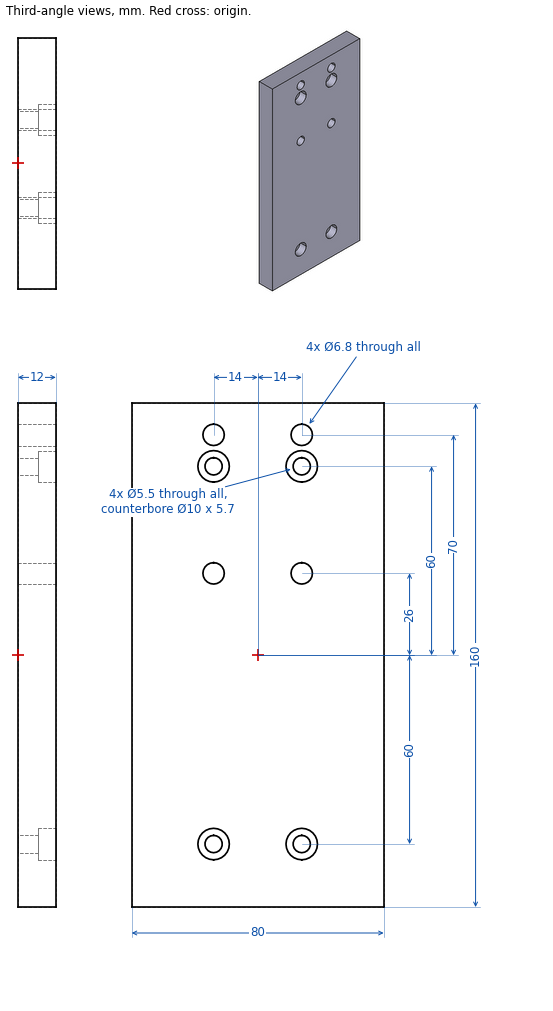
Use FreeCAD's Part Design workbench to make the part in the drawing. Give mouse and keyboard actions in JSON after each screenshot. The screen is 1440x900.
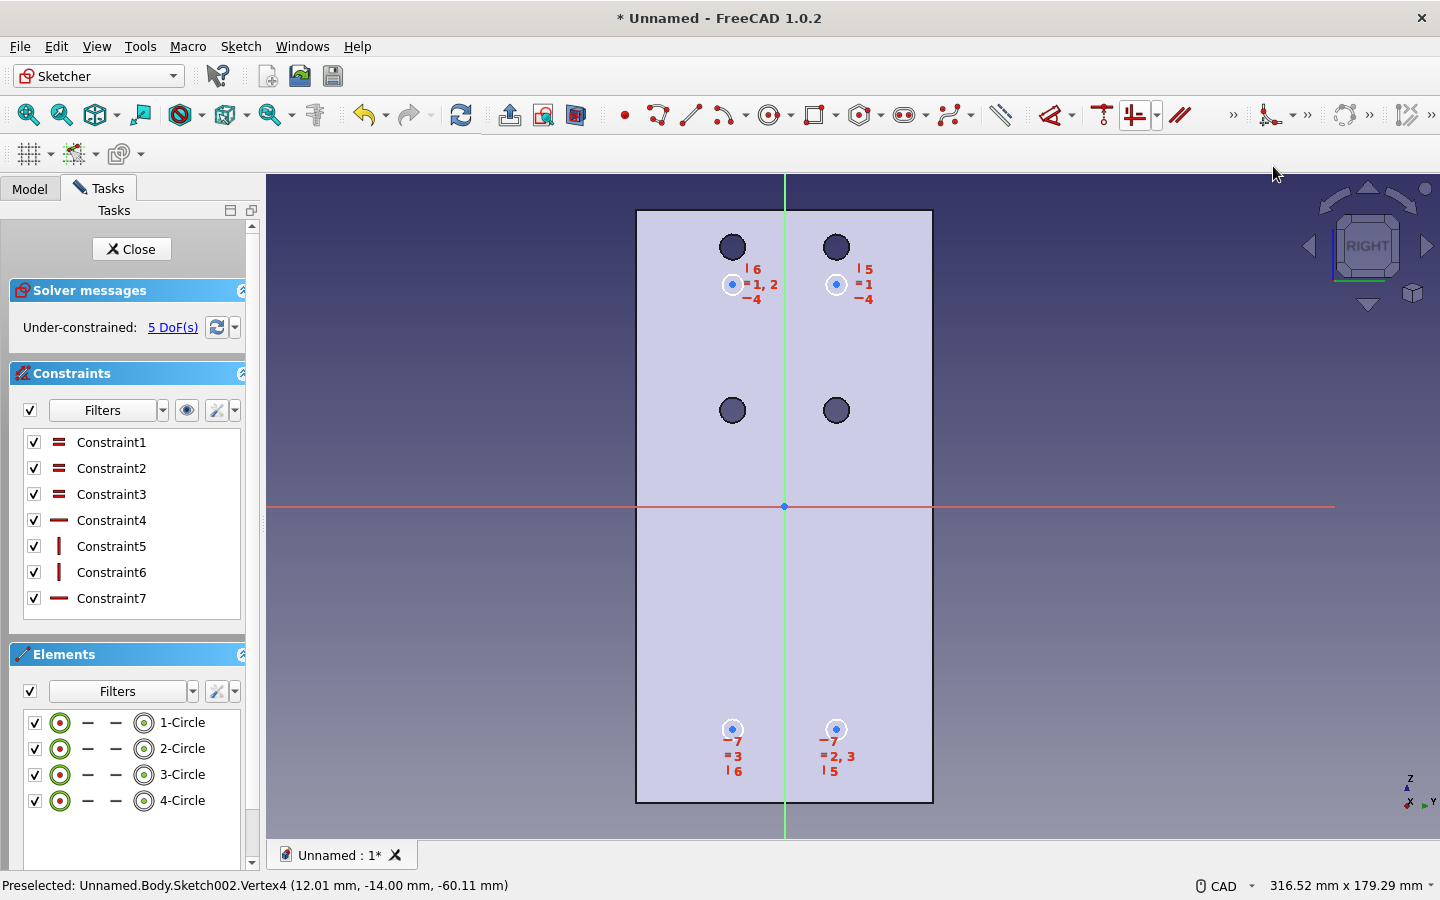
{"action": "left_click", "coordinate": [1050, 116]}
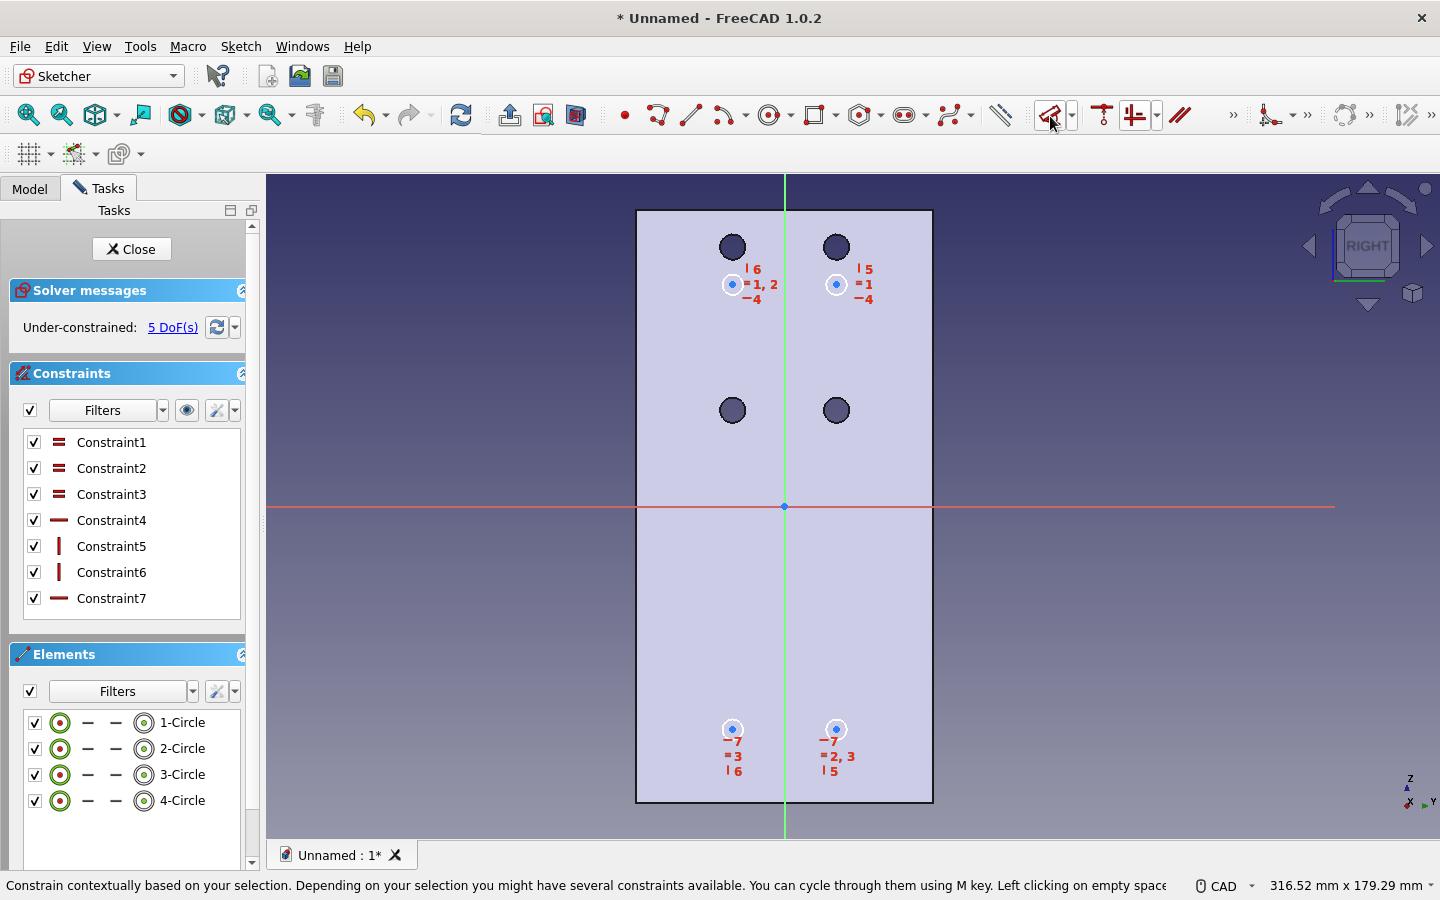
{"action": "scroll", "coordinate": [844, 278], "scroll_direction": "up", "scroll_amount": 4}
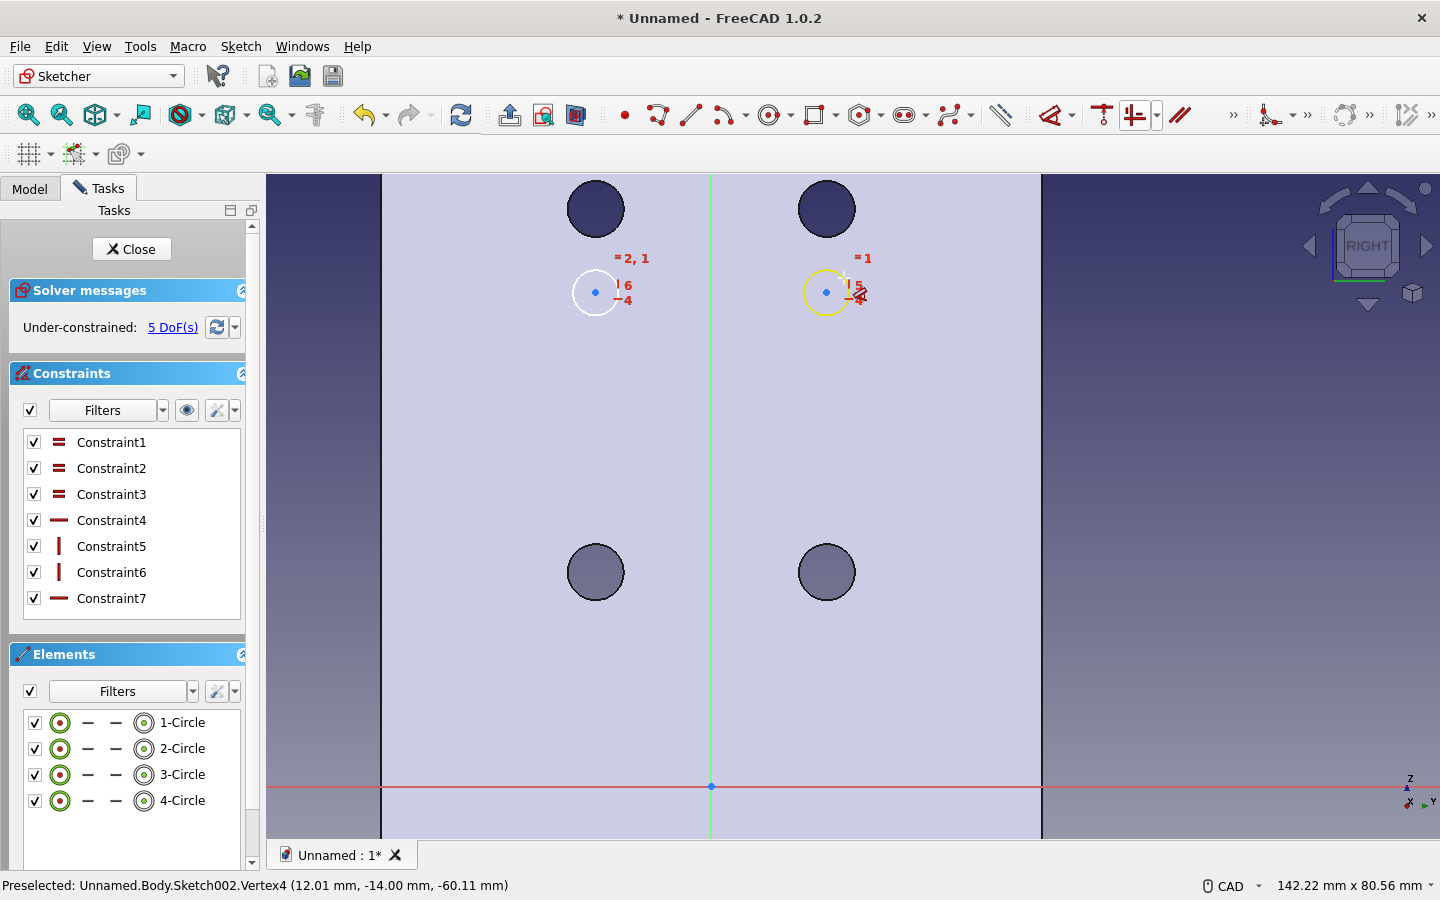
{"action": "left_click", "coordinate": [843, 277]}
{"action": "left_click", "coordinate": [866, 255]}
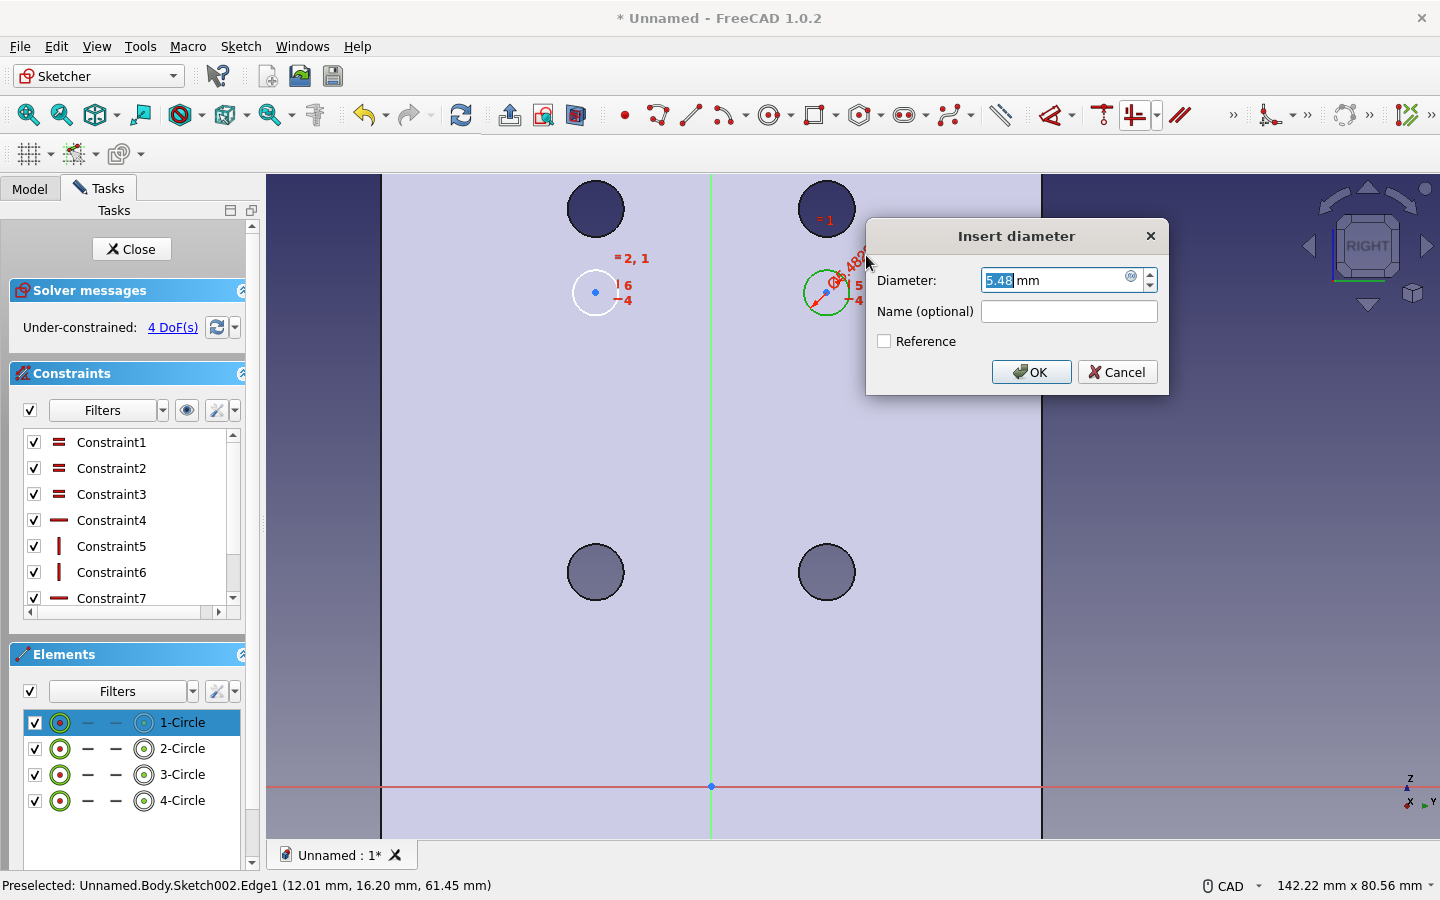
{"action": "type", "text": "5.5"}
{"action": "key", "text": "Return"}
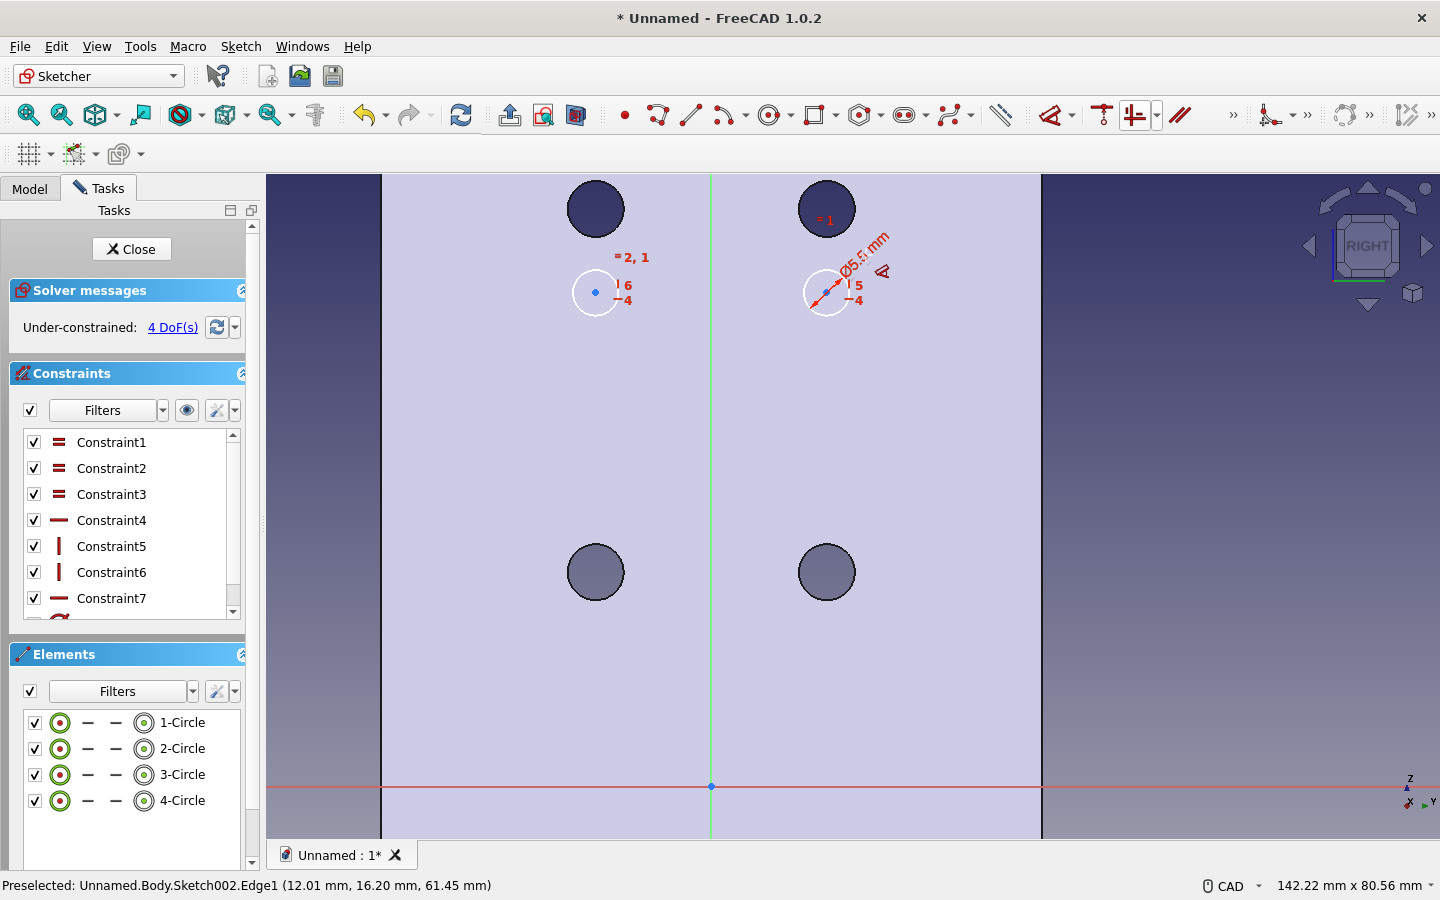
{"action": "left_click", "coordinate": [827, 293]}
{"action": "left_click", "coordinate": [769, 259]}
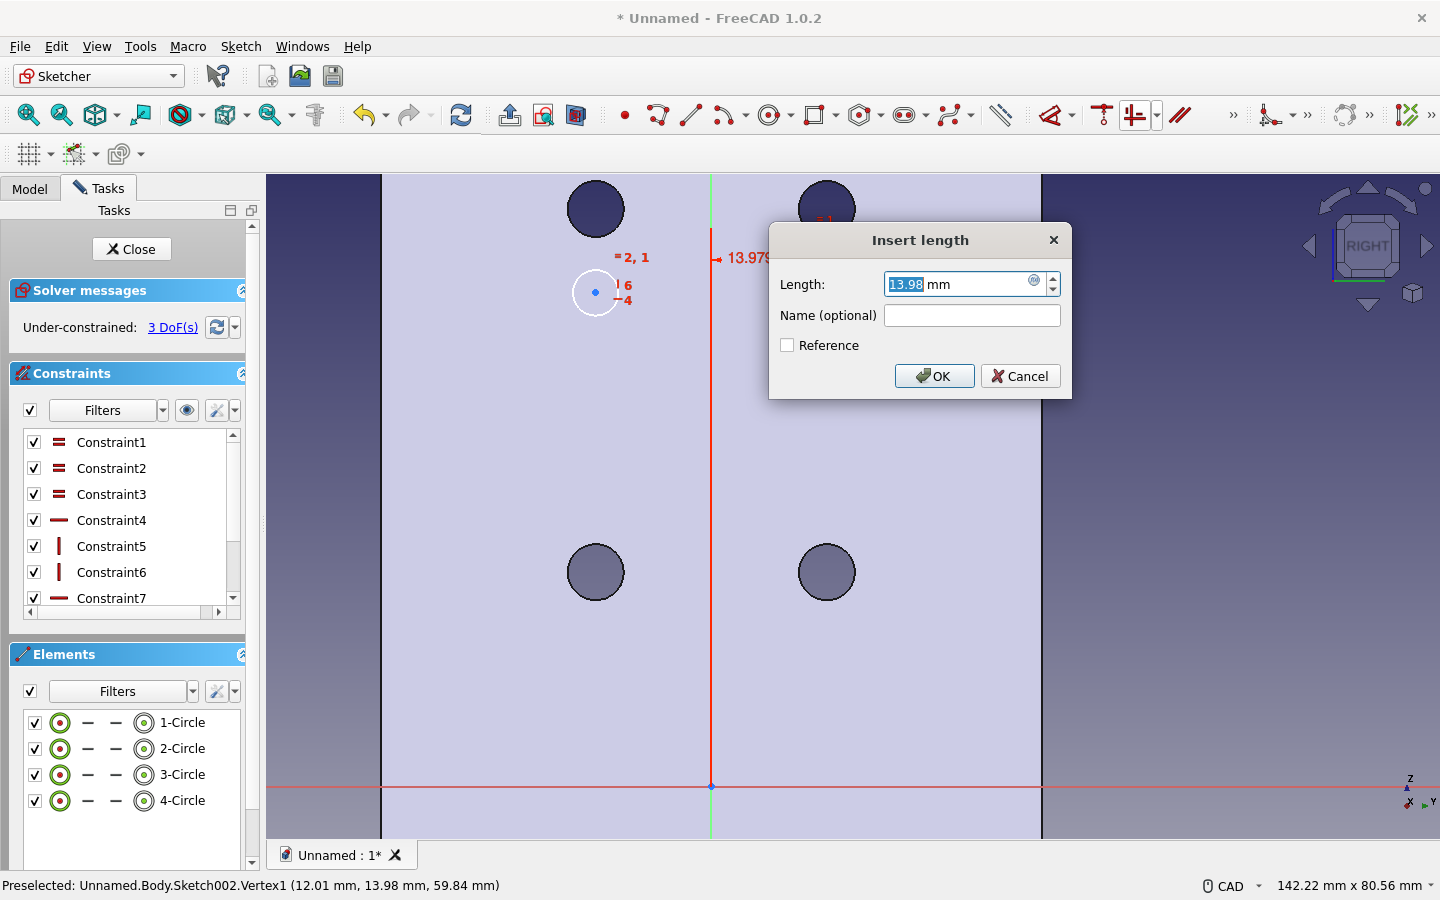
{"action": "type", "text": "14"}
{"action": "key", "text": "Return"}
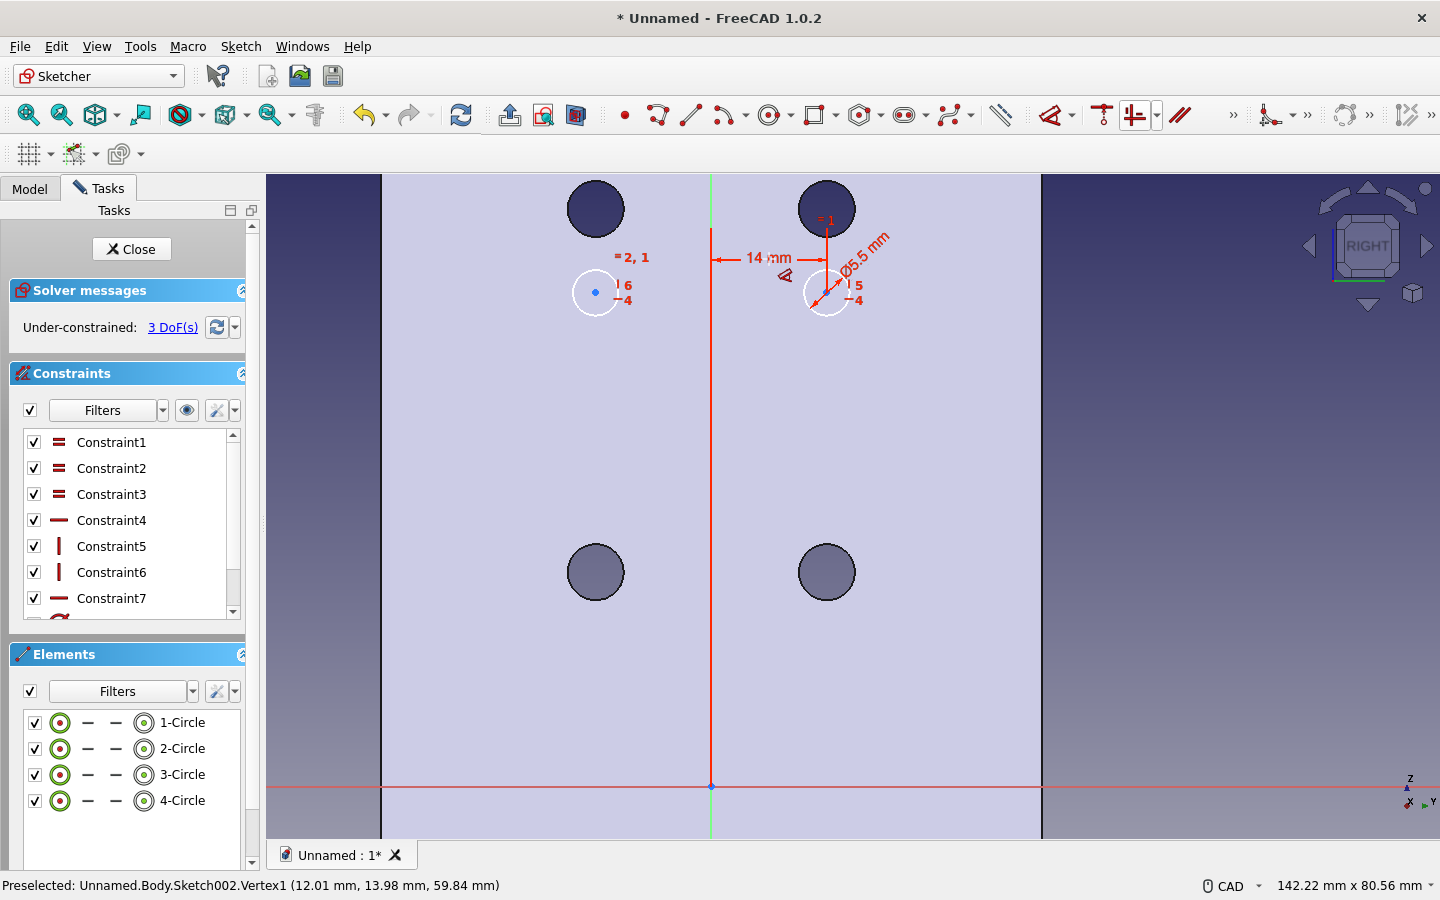
{"action": "left_click", "coordinate": [827, 293]}
{"action": "left_click", "coordinate": [861, 540]}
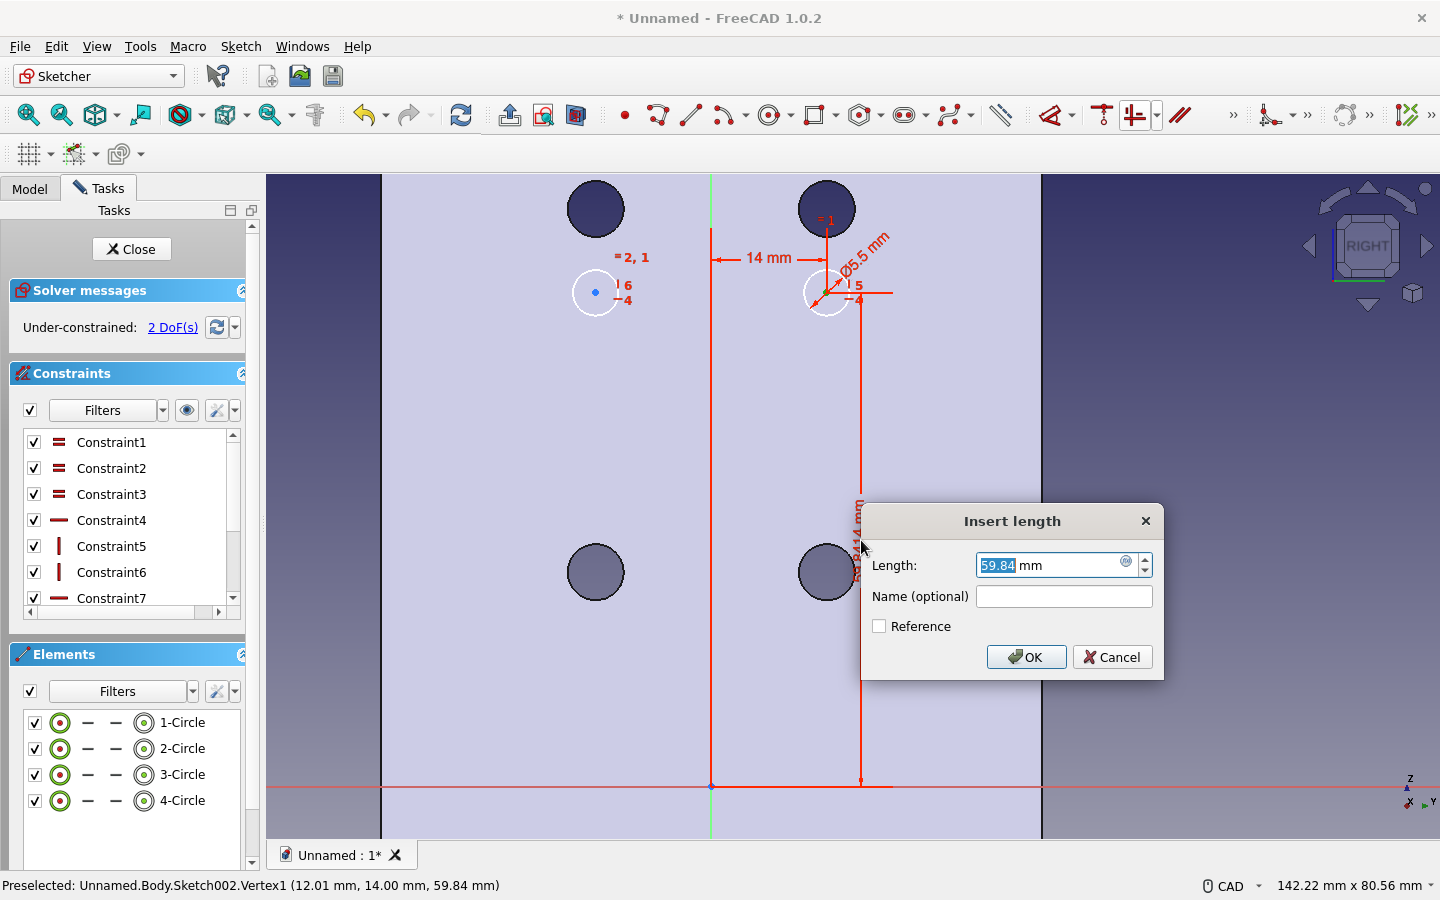
{"action": "type", "text": "60"}
{"action": "key", "text": "Return"}